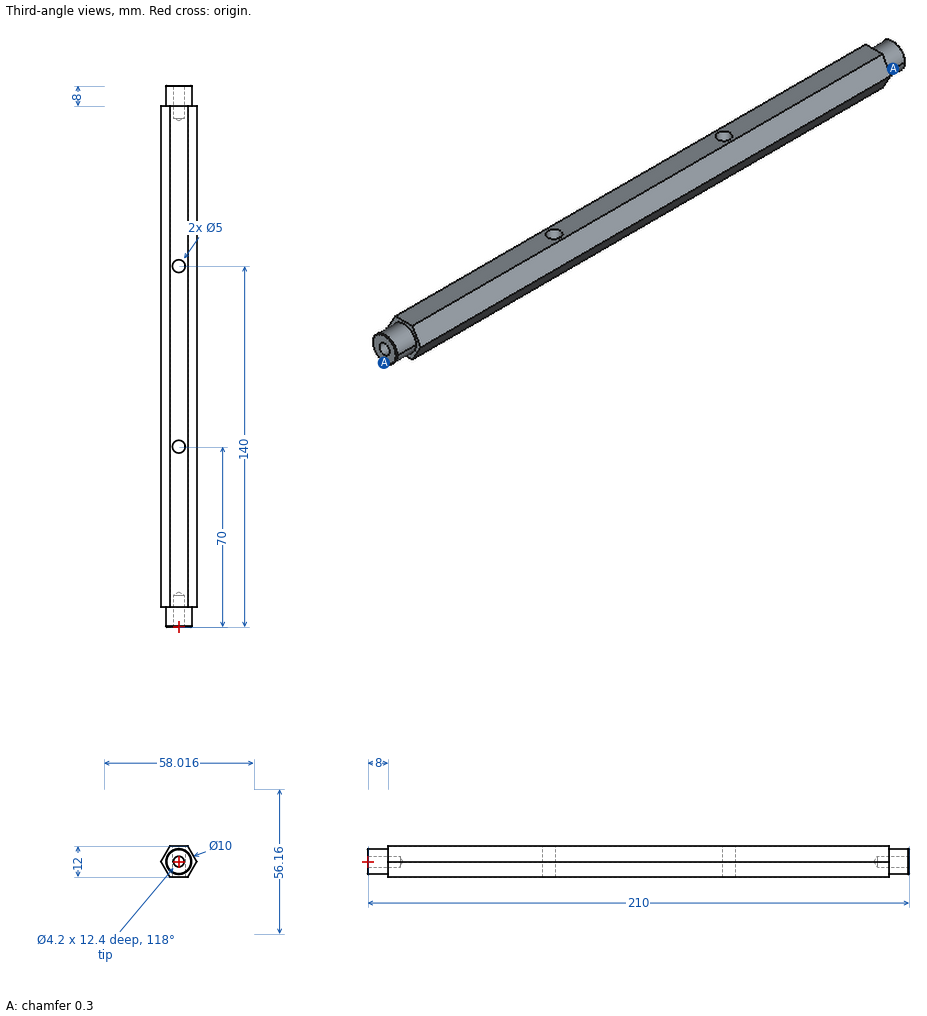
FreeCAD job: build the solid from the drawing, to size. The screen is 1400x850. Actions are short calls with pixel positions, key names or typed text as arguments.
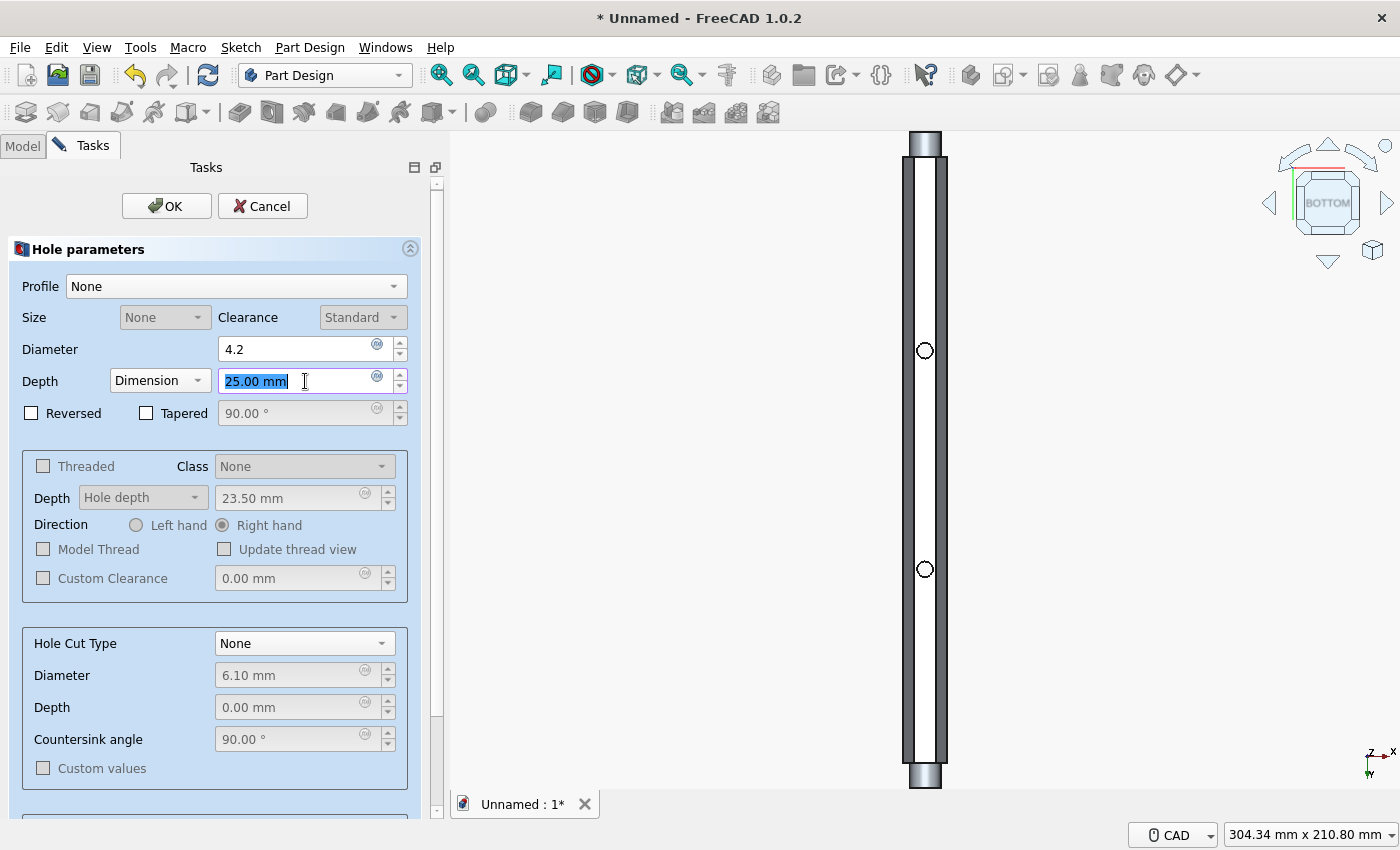
text(12.4)
key(Tab)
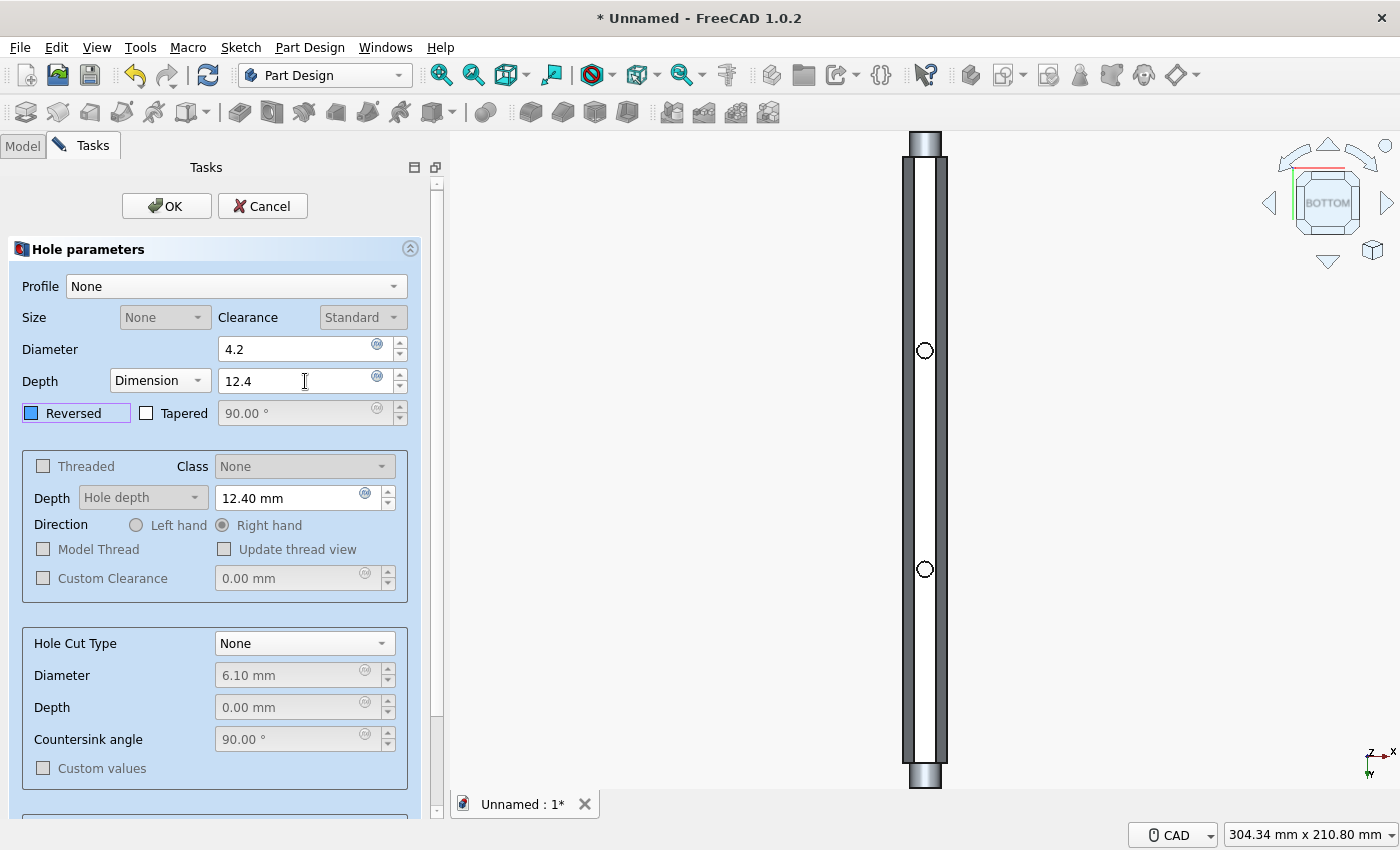
click(167, 206)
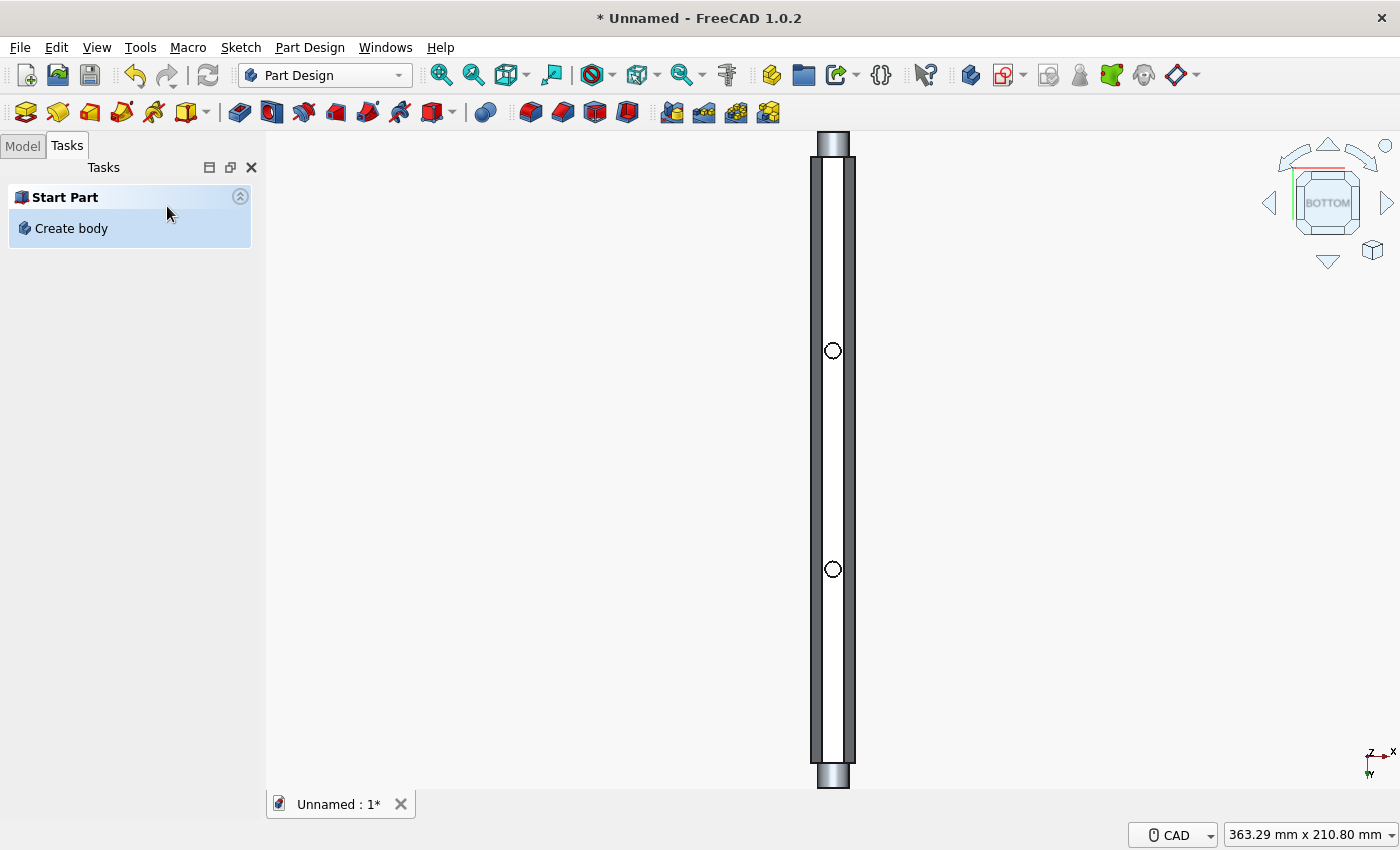
key(4)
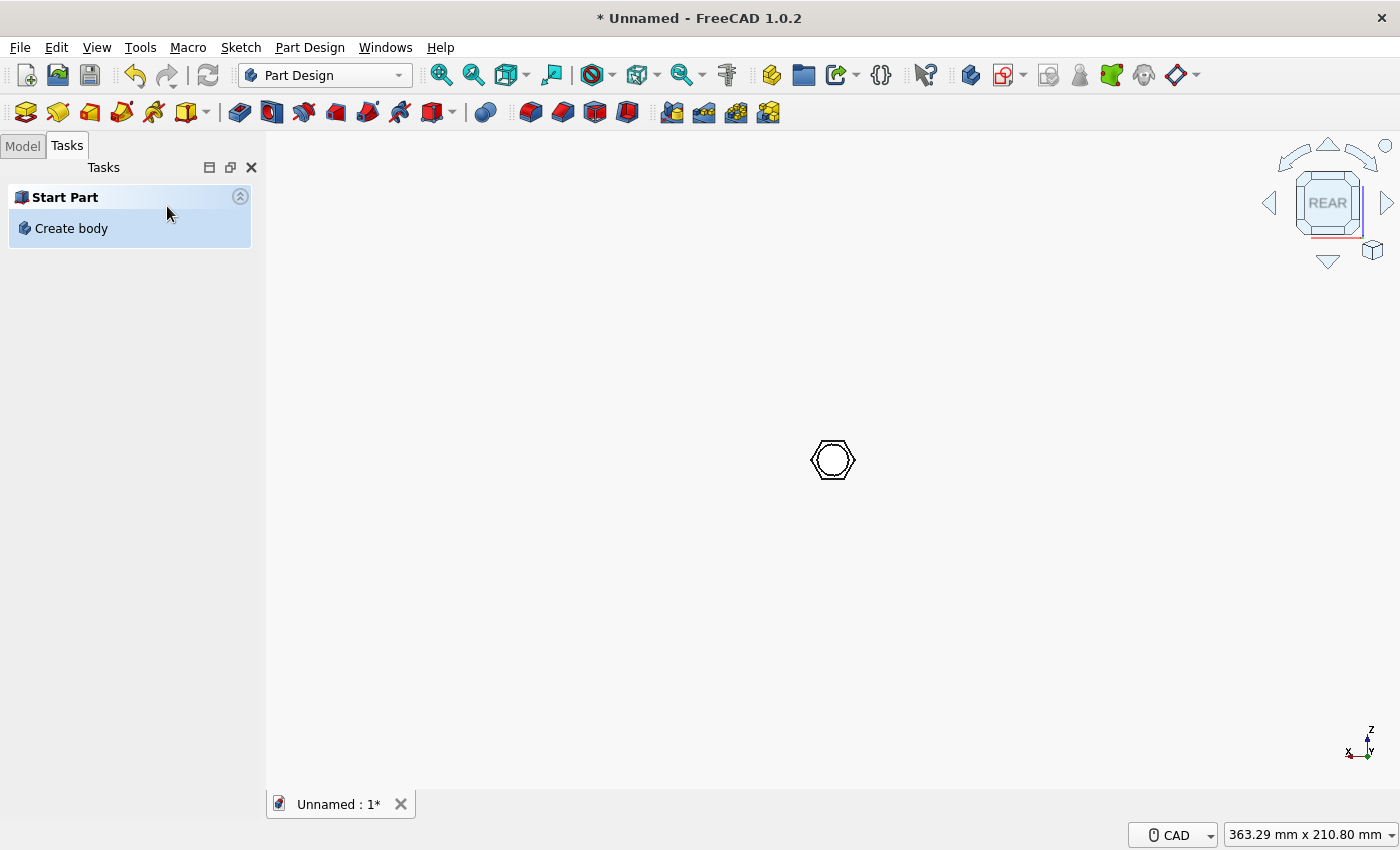
key(v)
key(f)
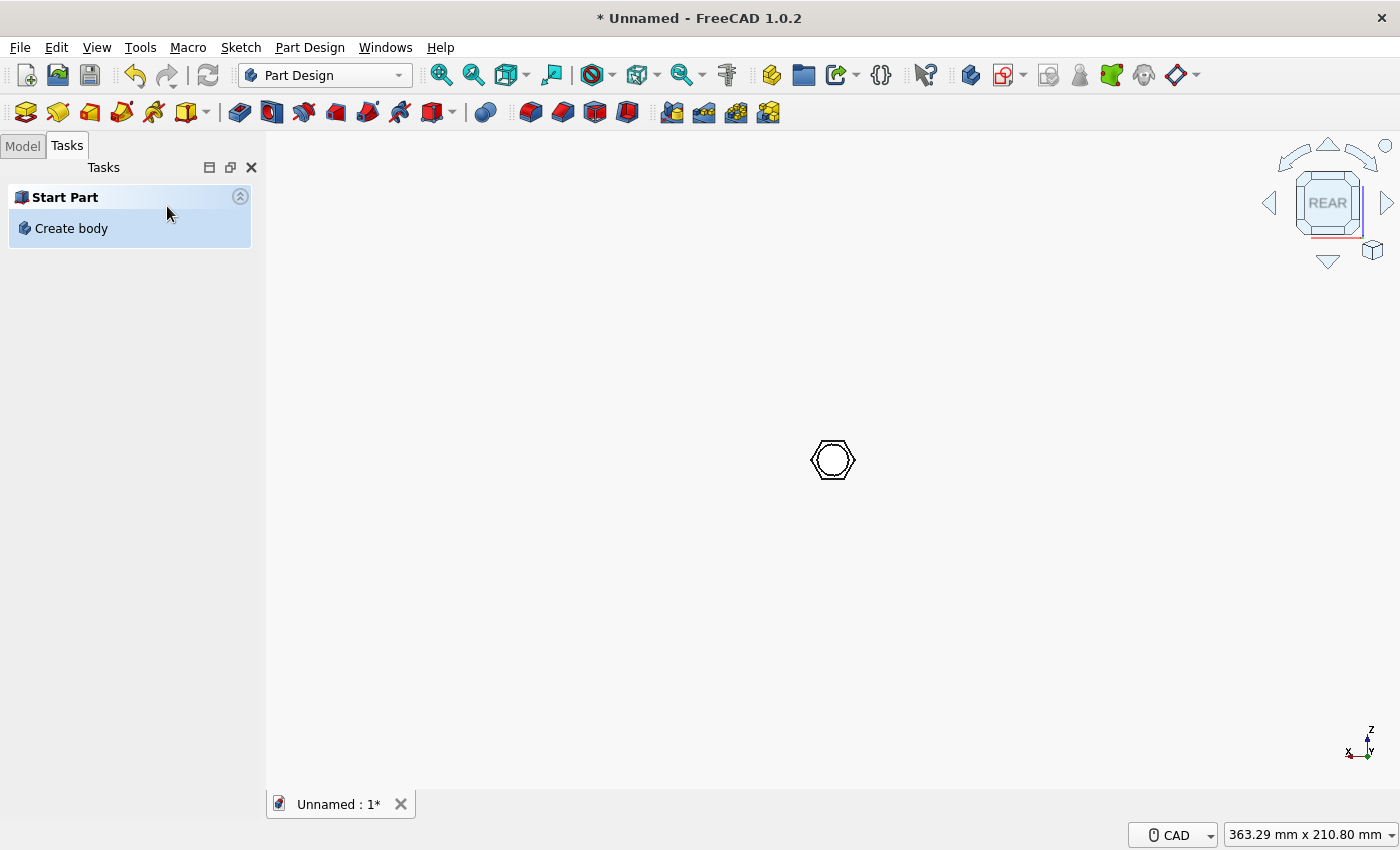
click(833, 459)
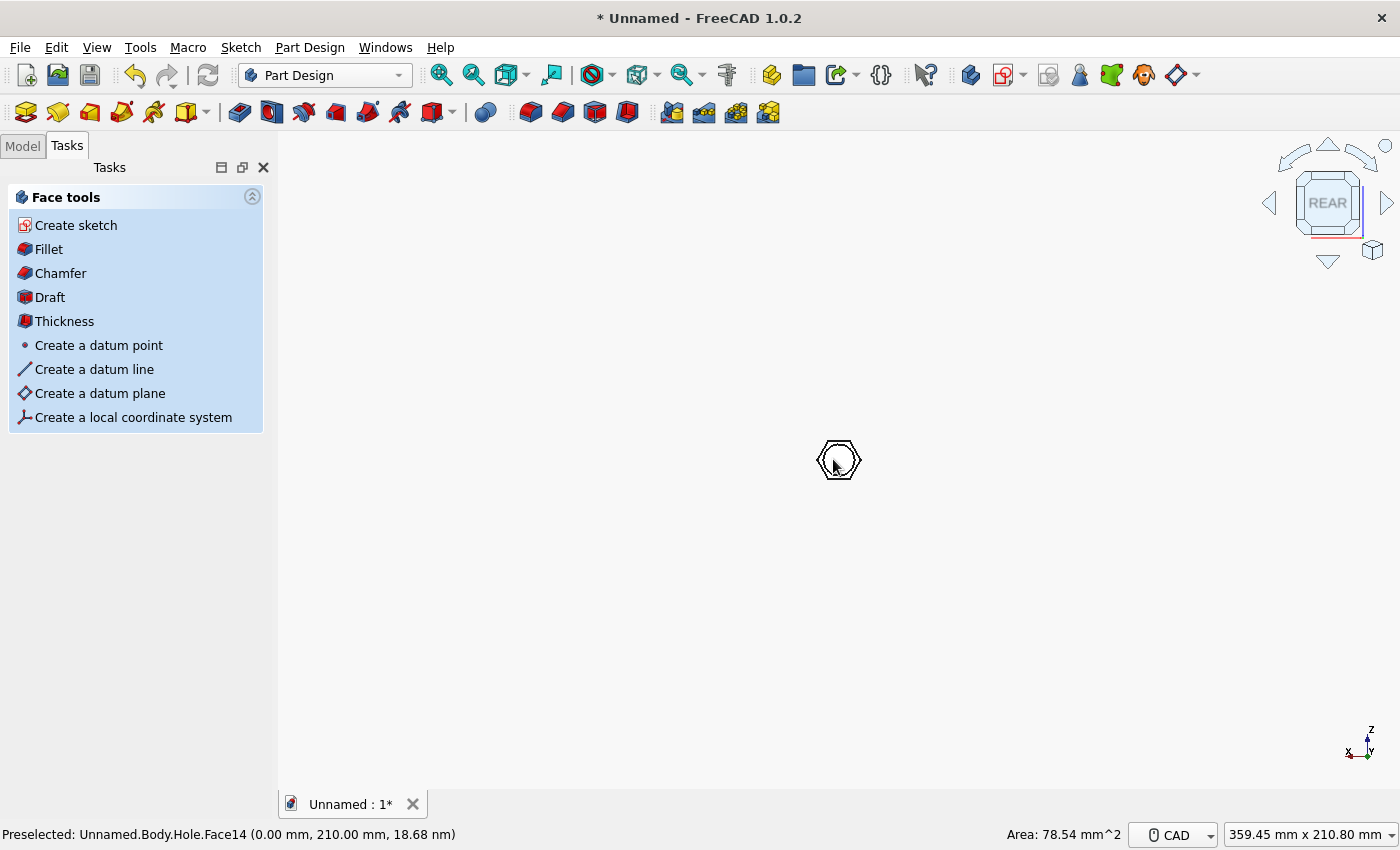
click(1004, 76)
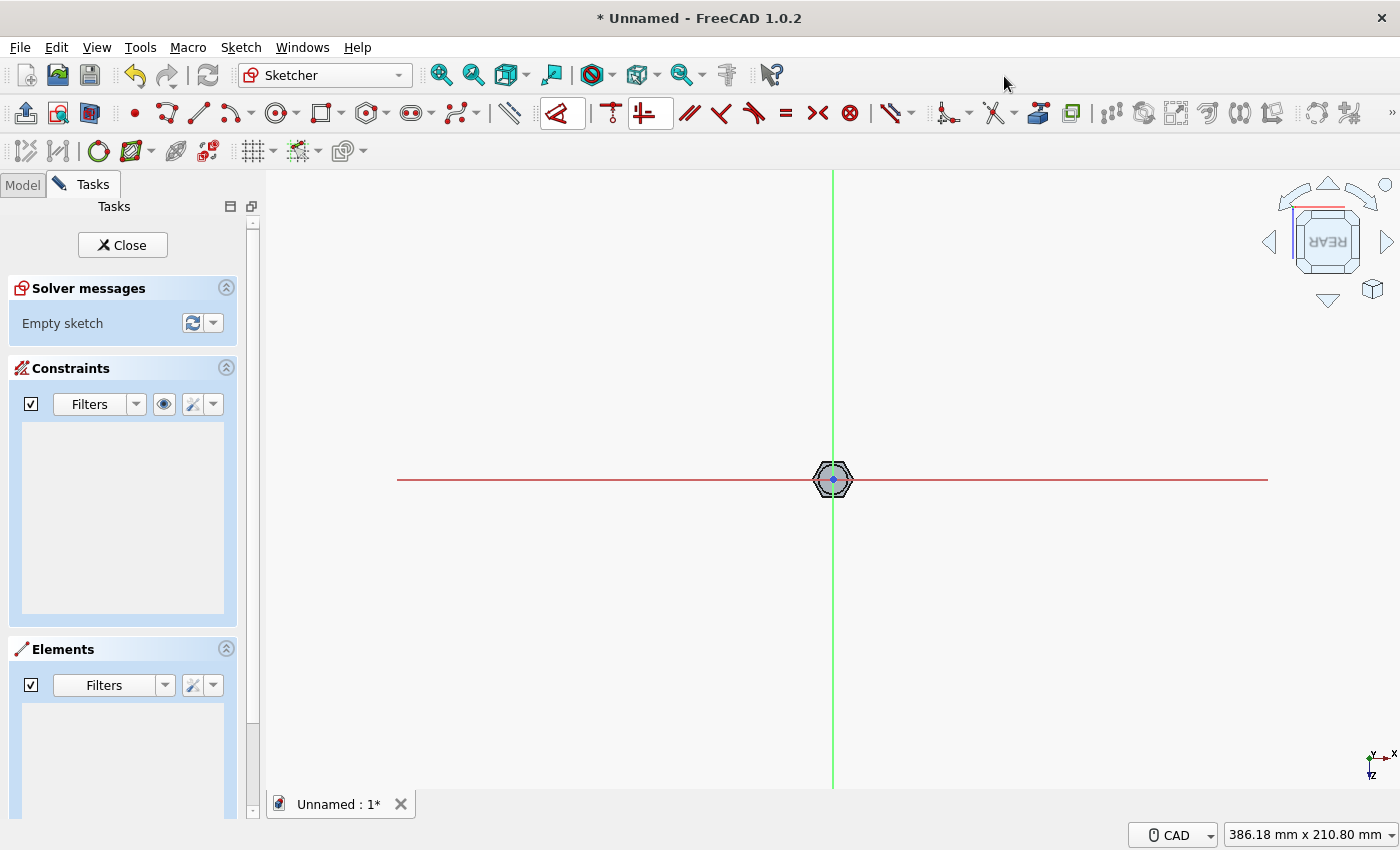
scroll(837, 479, up, 15)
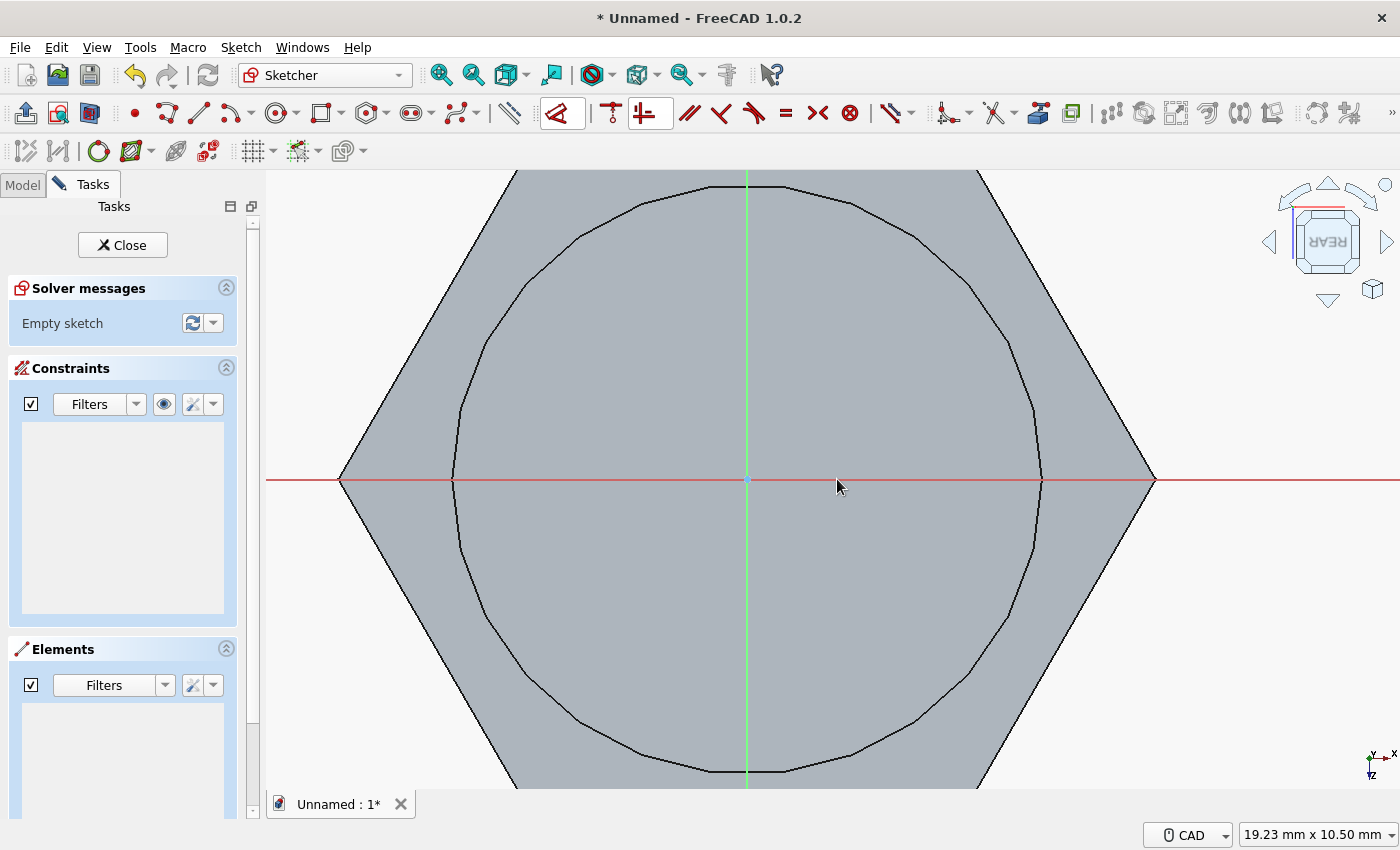
scroll(712, 479, up, 2)